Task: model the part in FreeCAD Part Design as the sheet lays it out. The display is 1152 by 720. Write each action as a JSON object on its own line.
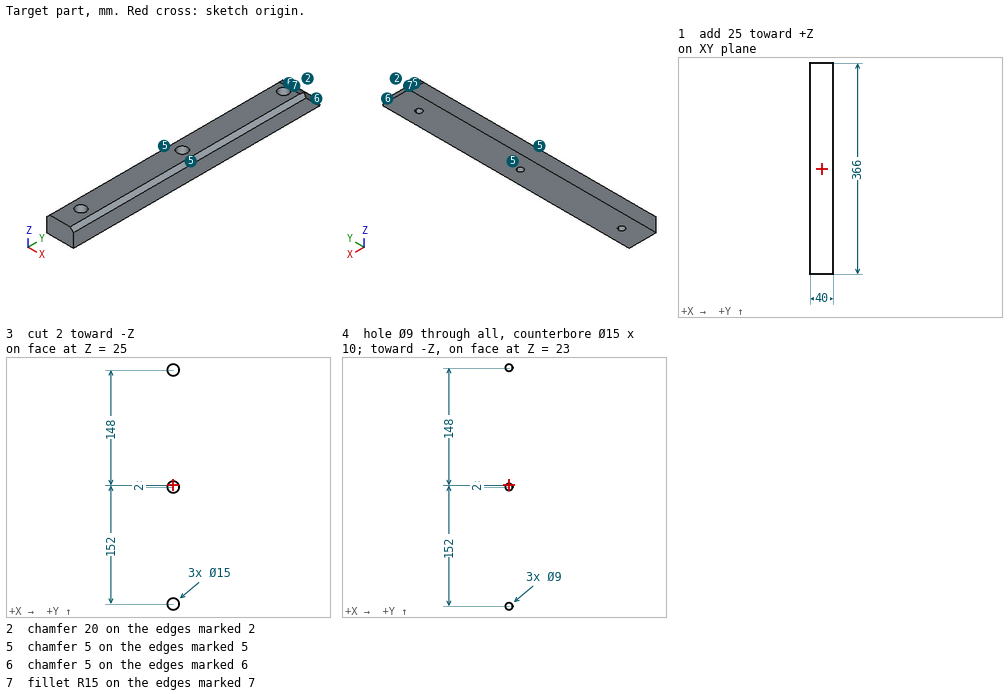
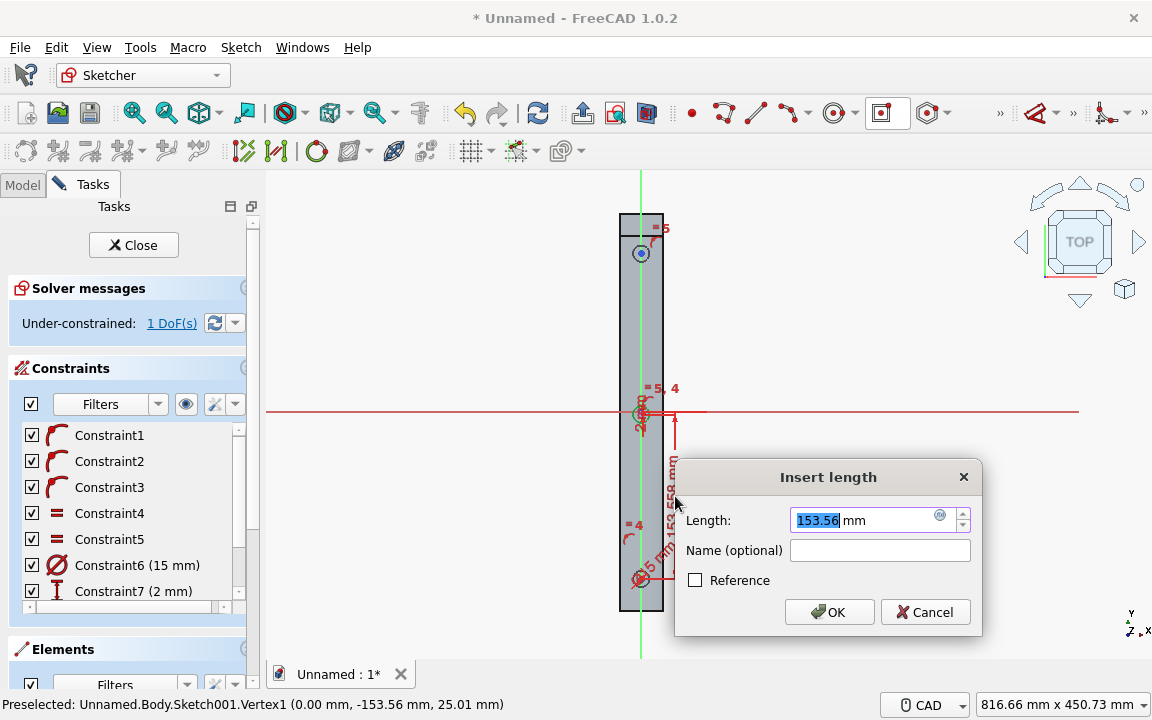
{"action": "type", "text": "152"}
{"action": "key", "text": "Return"}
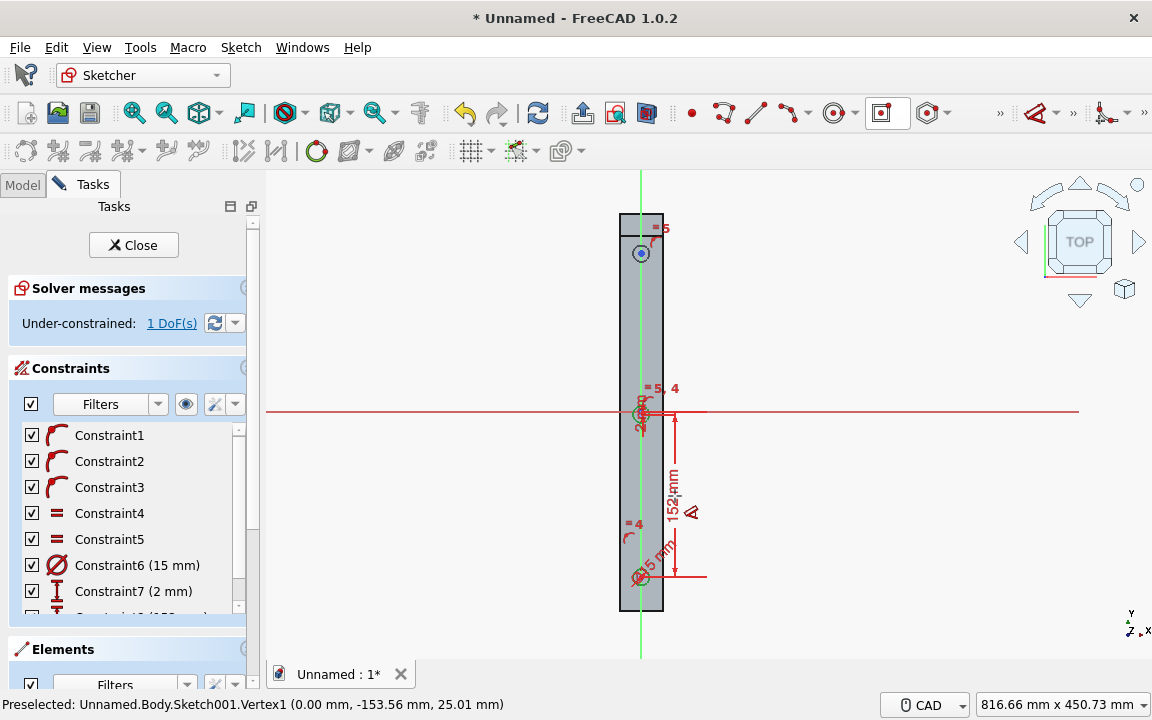
{"action": "left_click", "coordinate": [641, 254]}
{"action": "left_click", "coordinate": [675, 333]}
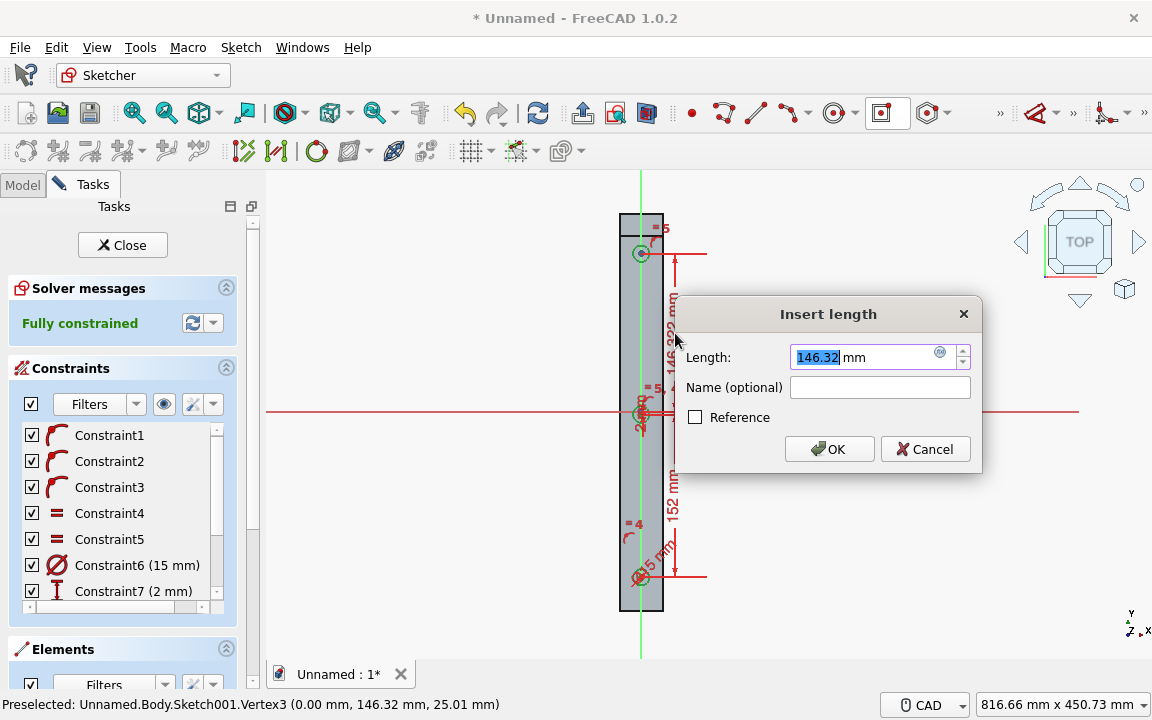
{"action": "type", "text": "148"}
{"action": "key", "text": "Return"}
{"action": "key", "text": "Escape"}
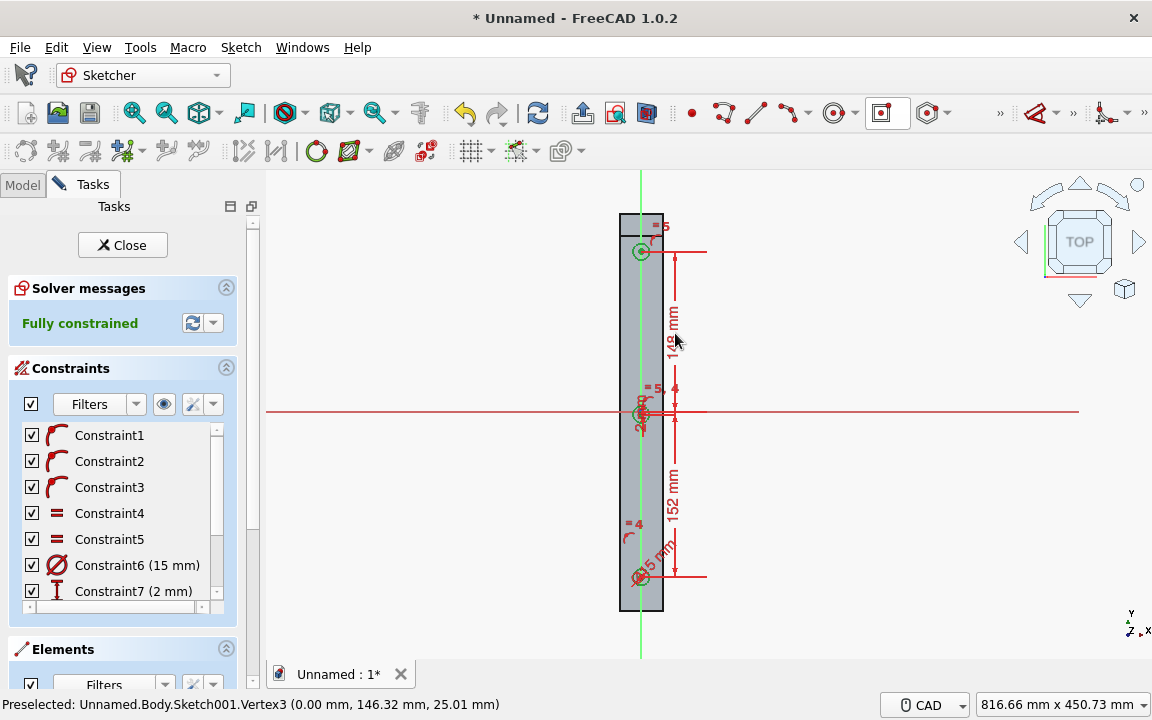
{"action": "left_click", "coordinate": [123, 245]}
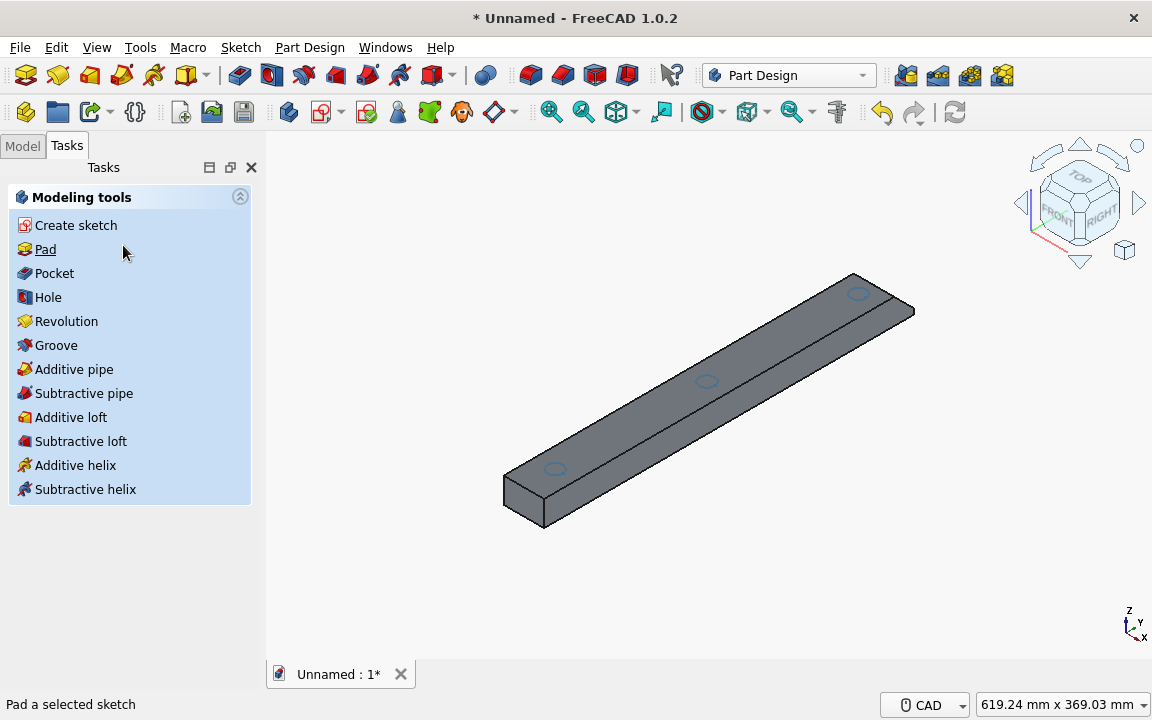
{"action": "left_click", "coordinate": [240, 76]}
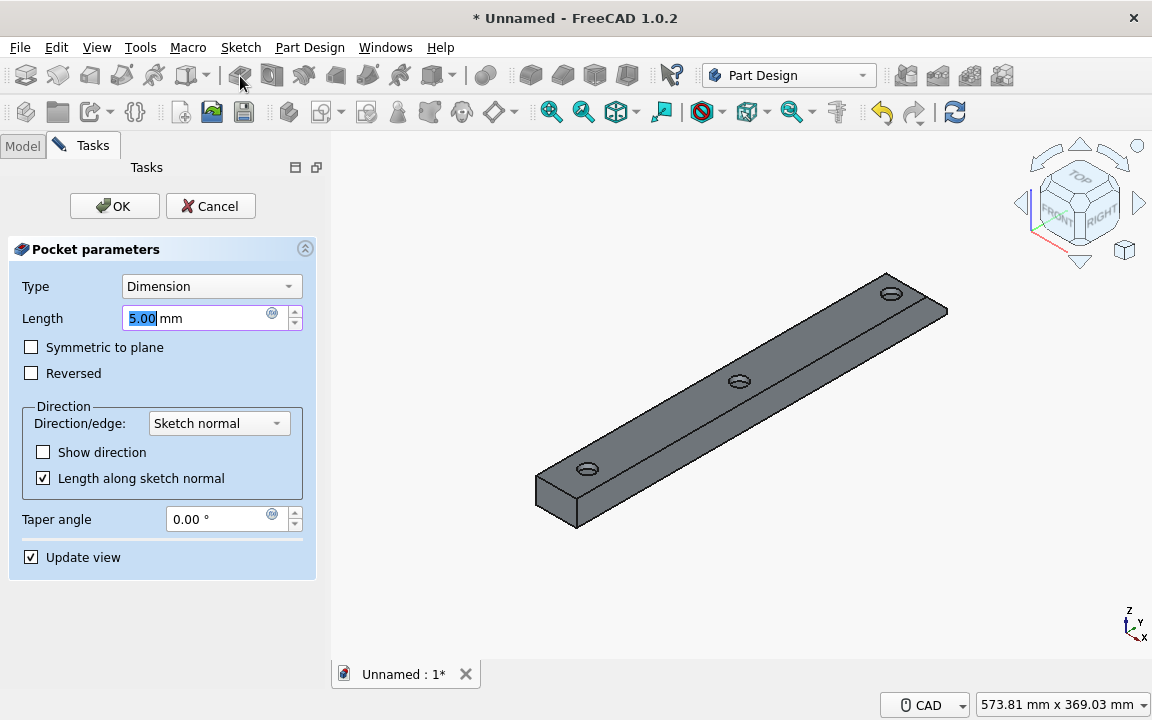
{"action": "type", "text": "2"}
{"action": "key", "text": "Tab"}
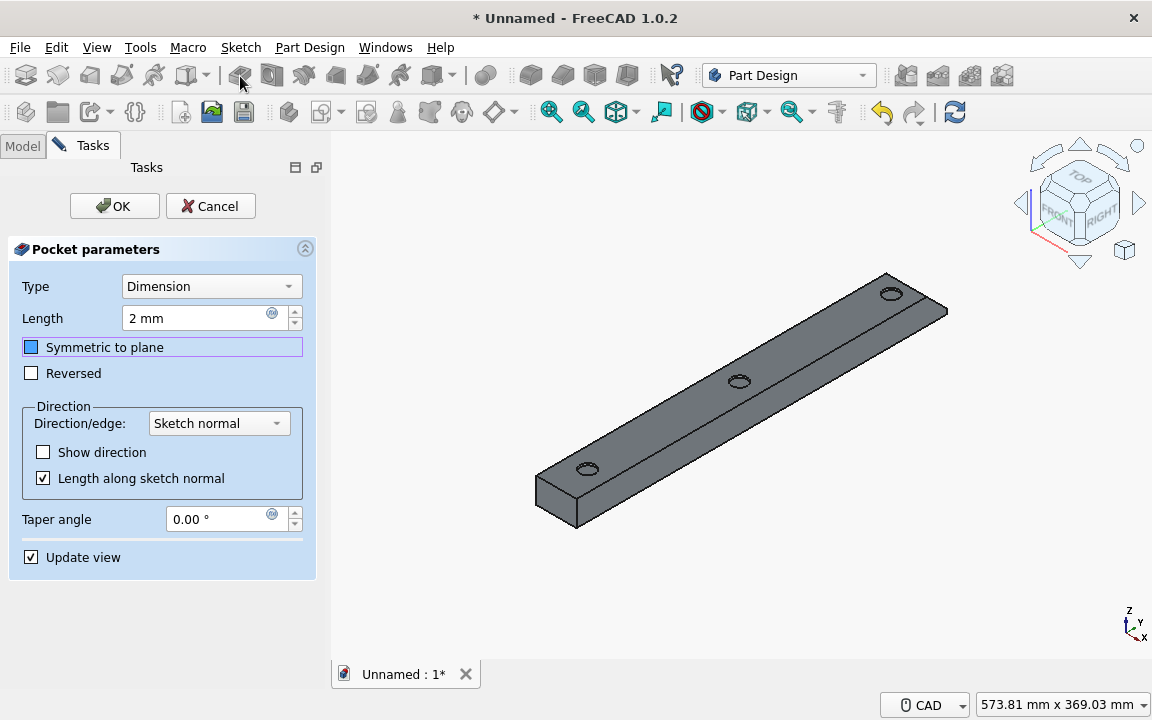
{"action": "left_click", "coordinate": [115, 206]}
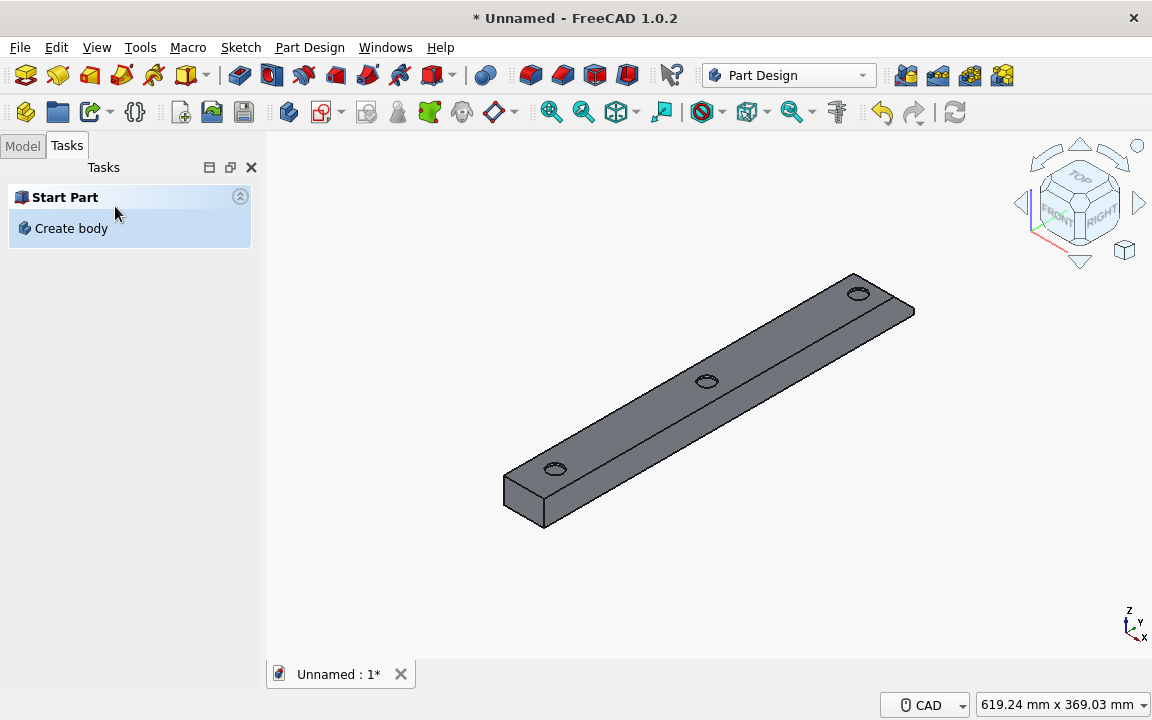
{"action": "key", "text": "2"}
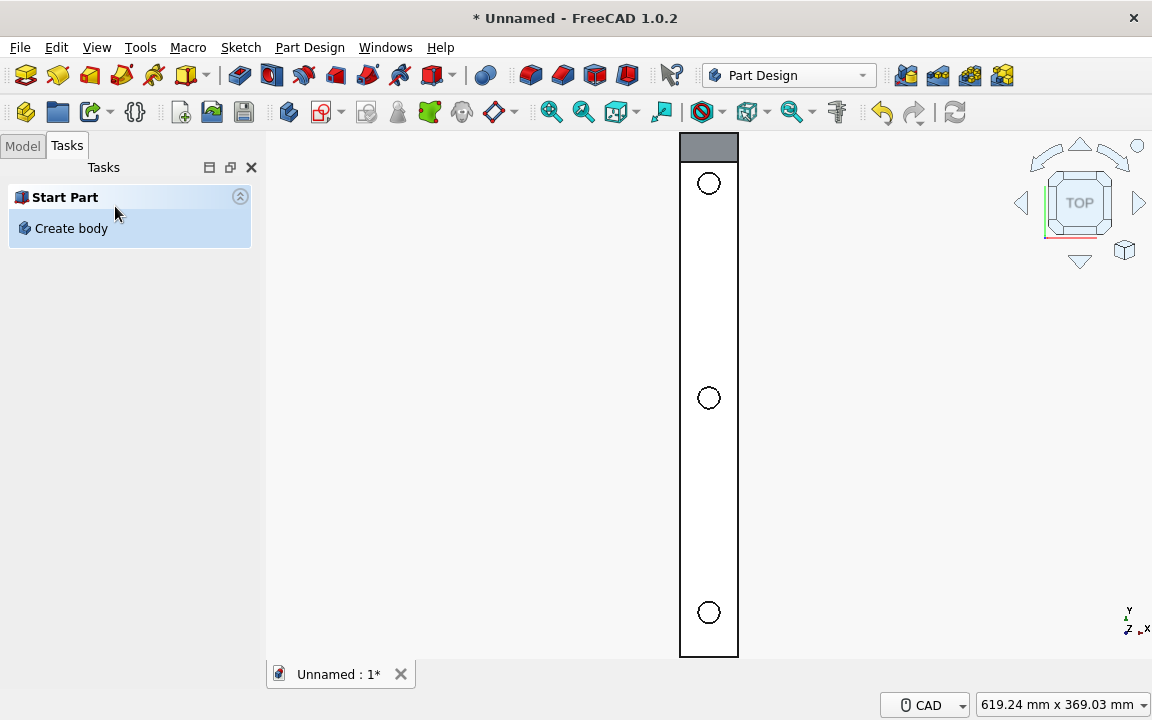
{"action": "left_click", "coordinate": [709, 182]}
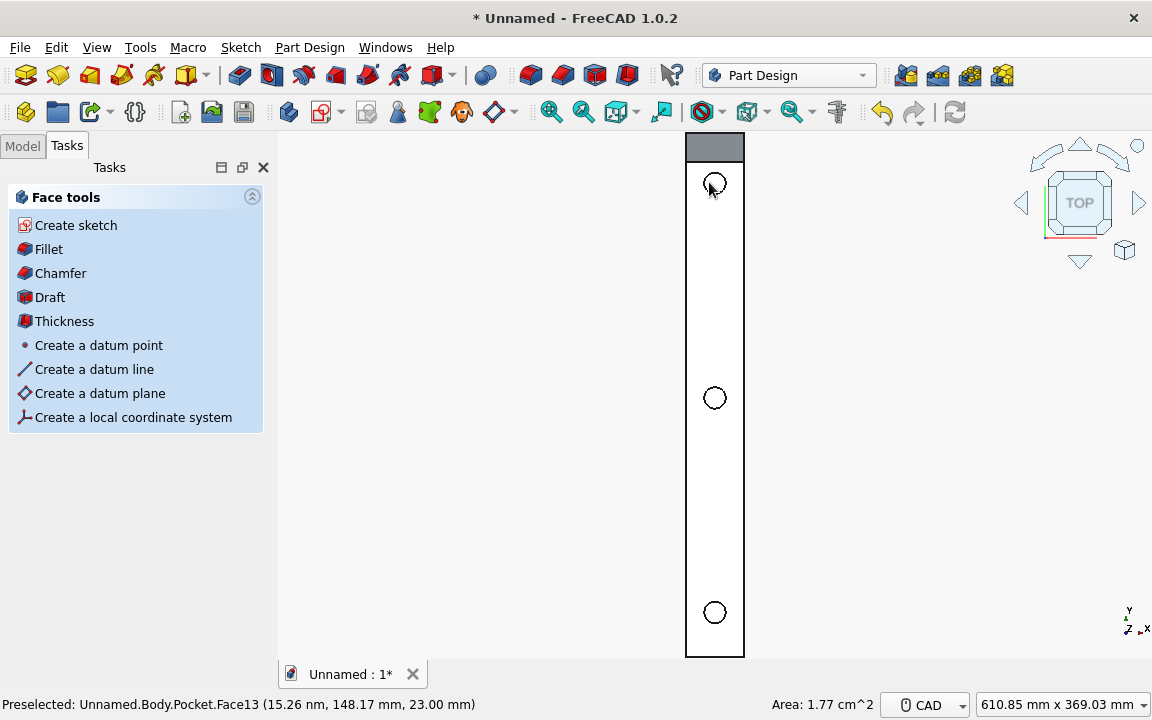
{"action": "left_click", "coordinate": [322, 112]}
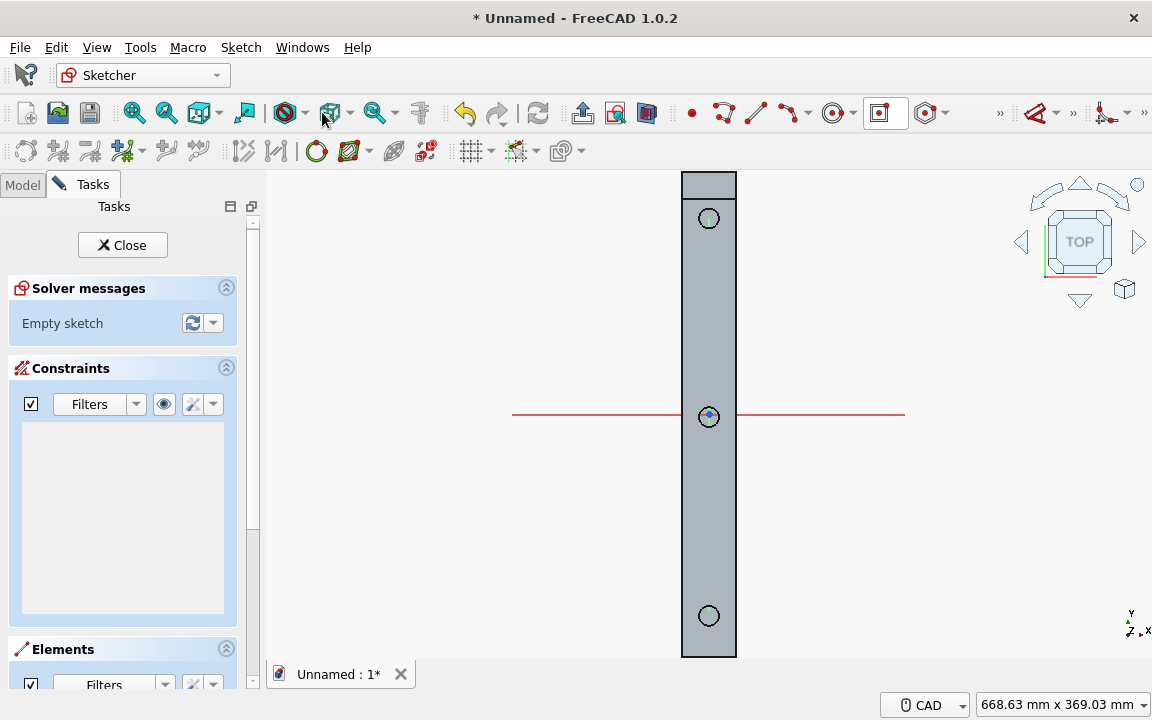
{"action": "left_click", "coordinate": [648, 114]}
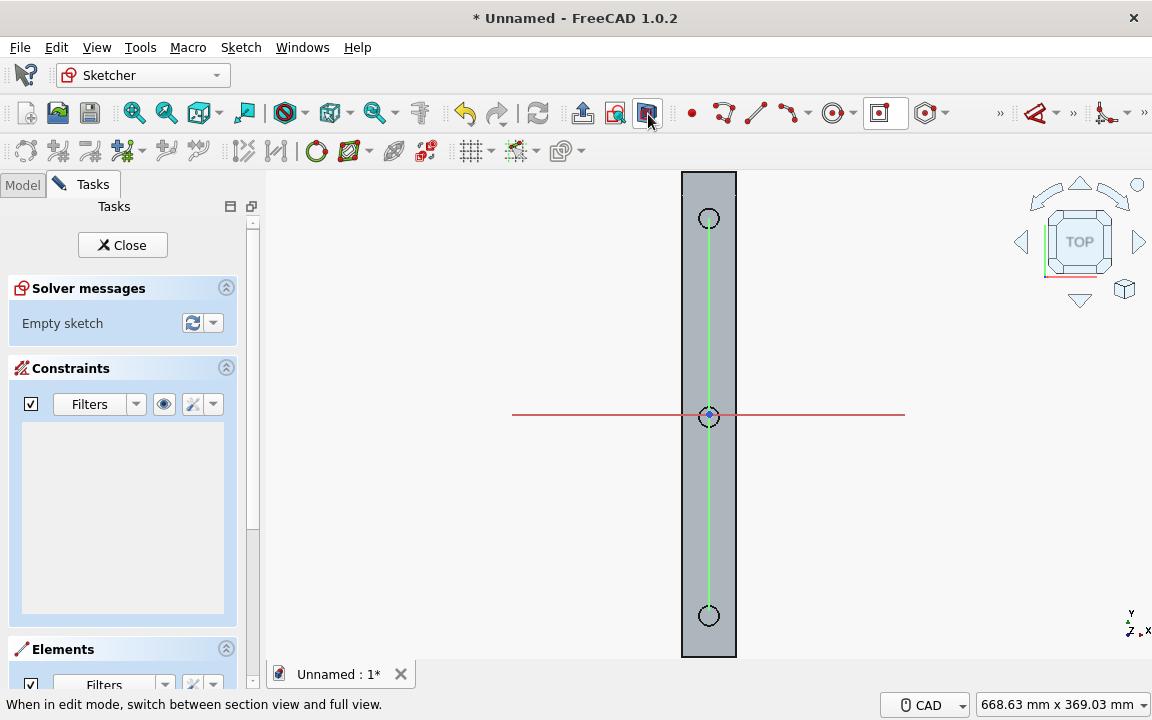
{"action": "scroll", "coordinate": [331, 403], "scroll_direction": "down", "scroll_amount": 1}